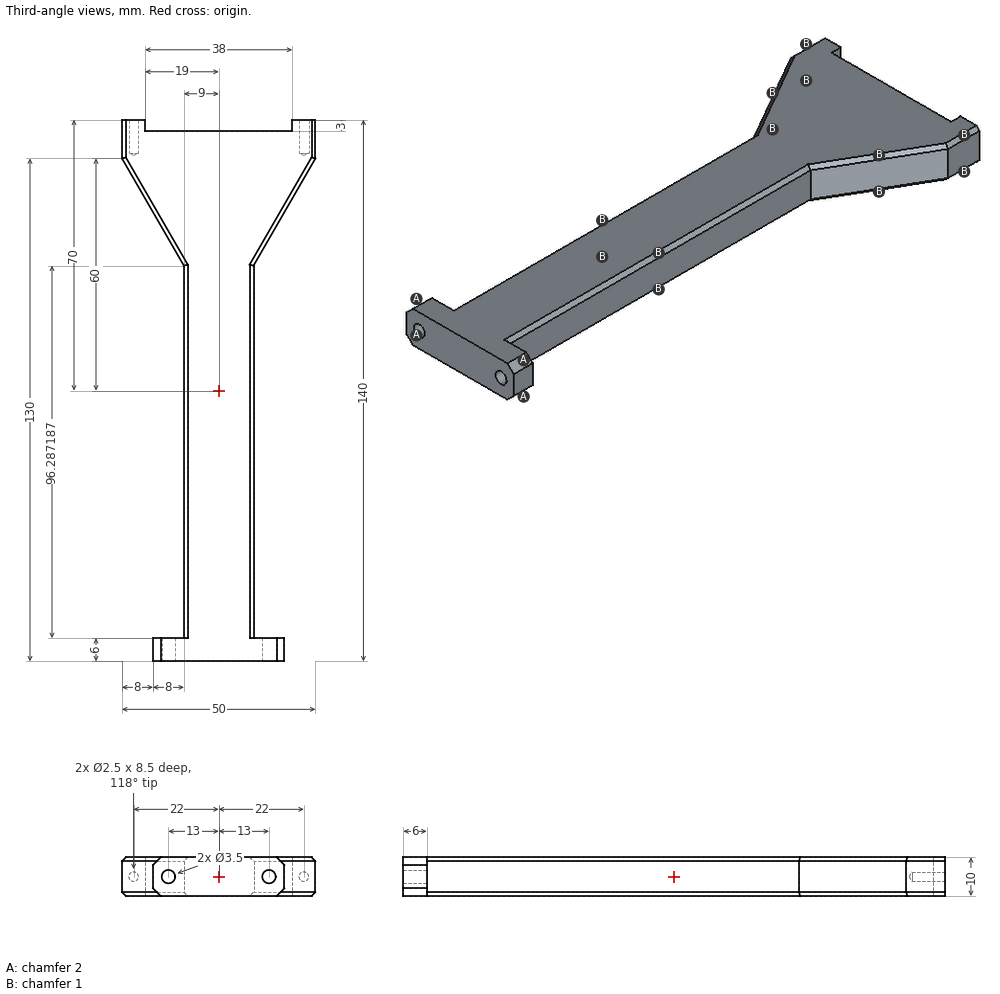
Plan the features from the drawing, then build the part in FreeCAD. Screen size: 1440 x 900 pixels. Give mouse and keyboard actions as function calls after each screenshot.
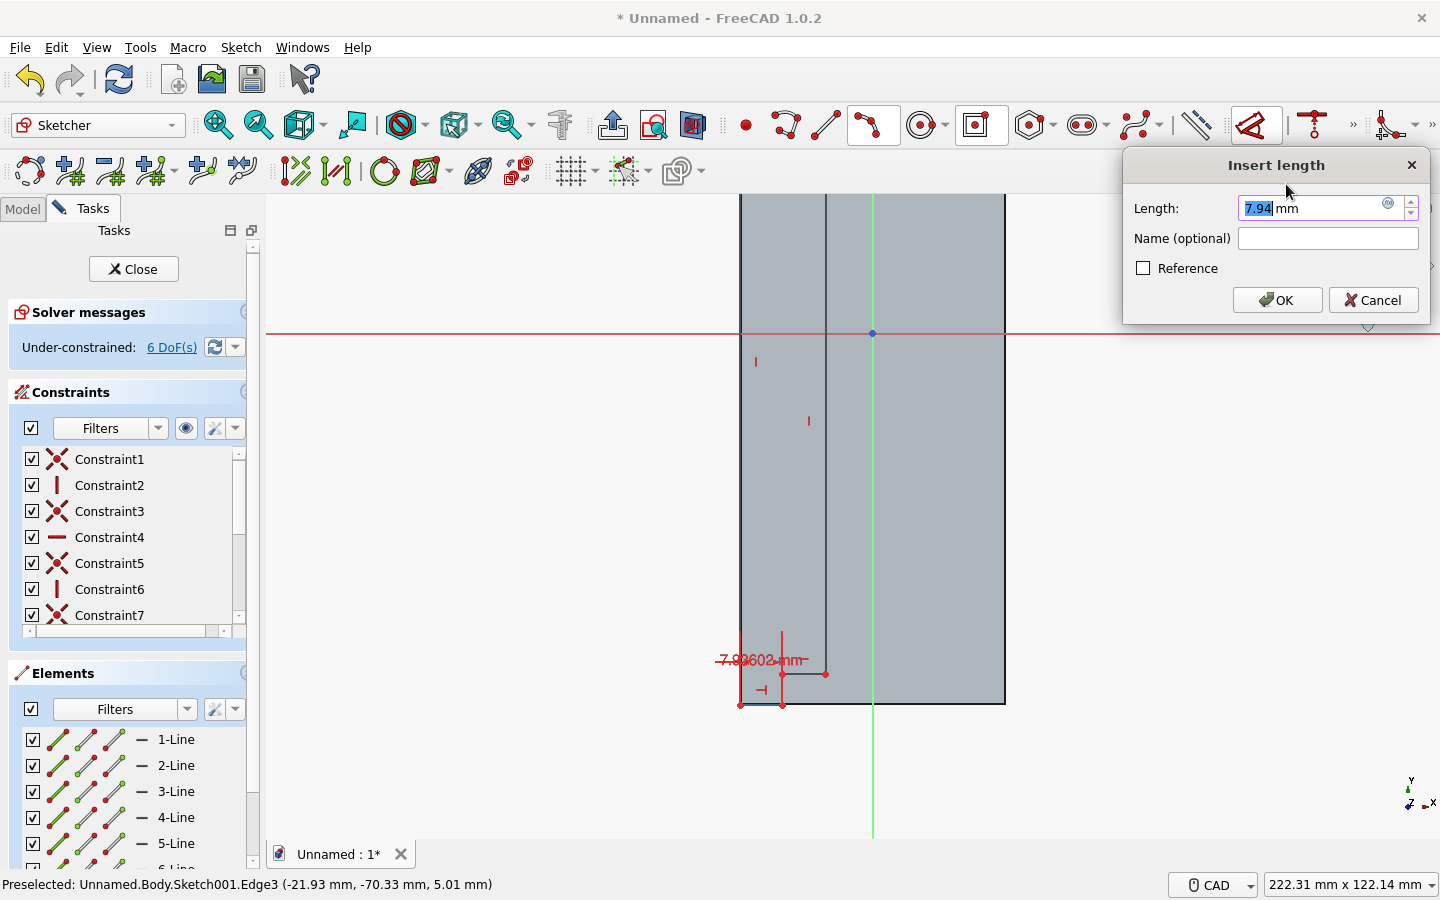
text(8)
key(Return)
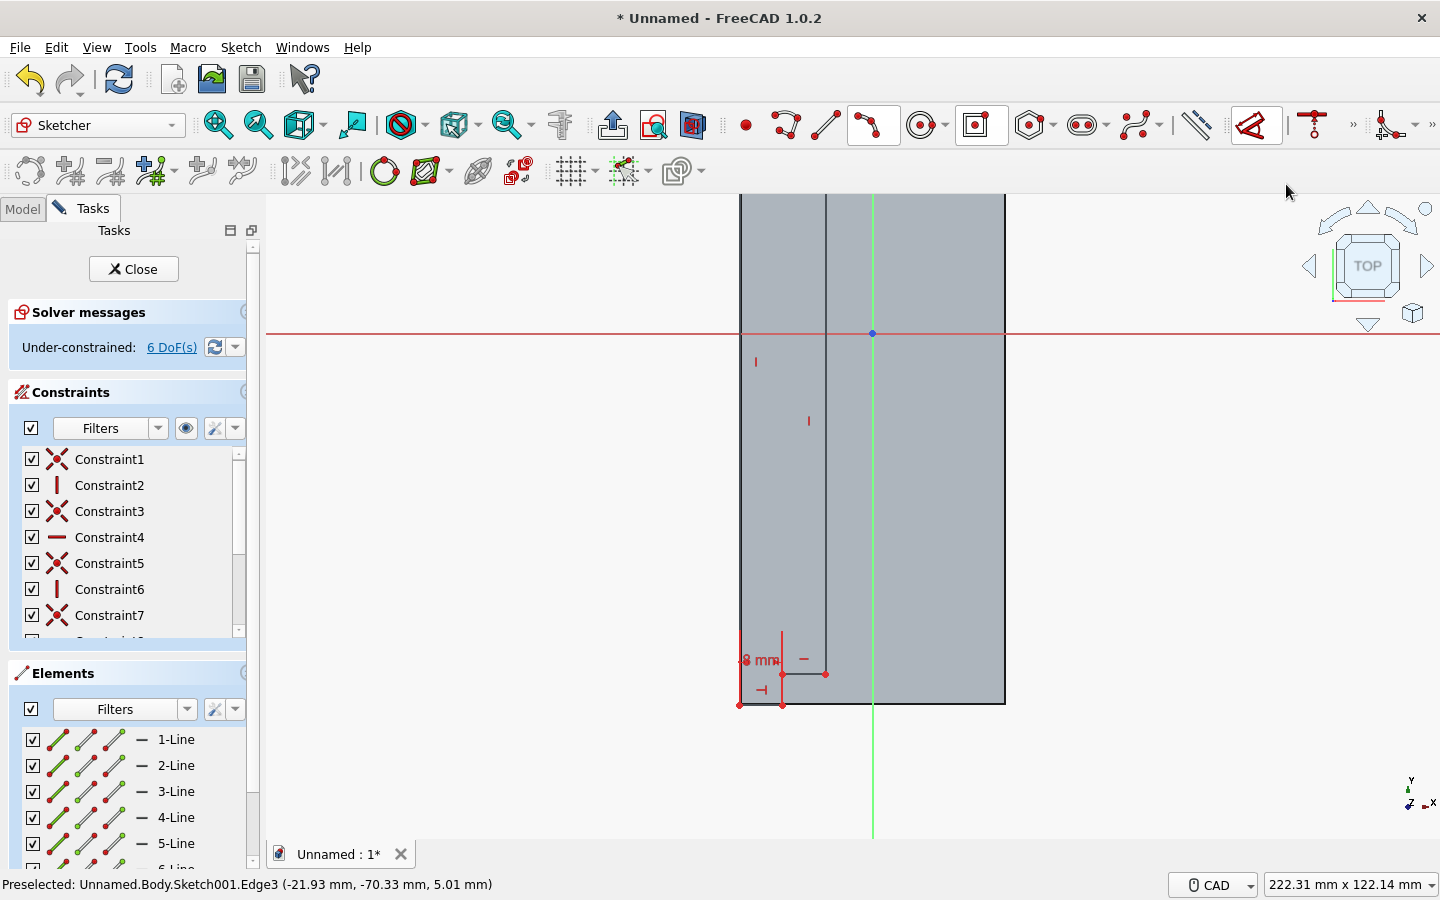
scroll(782, 696, up, 2)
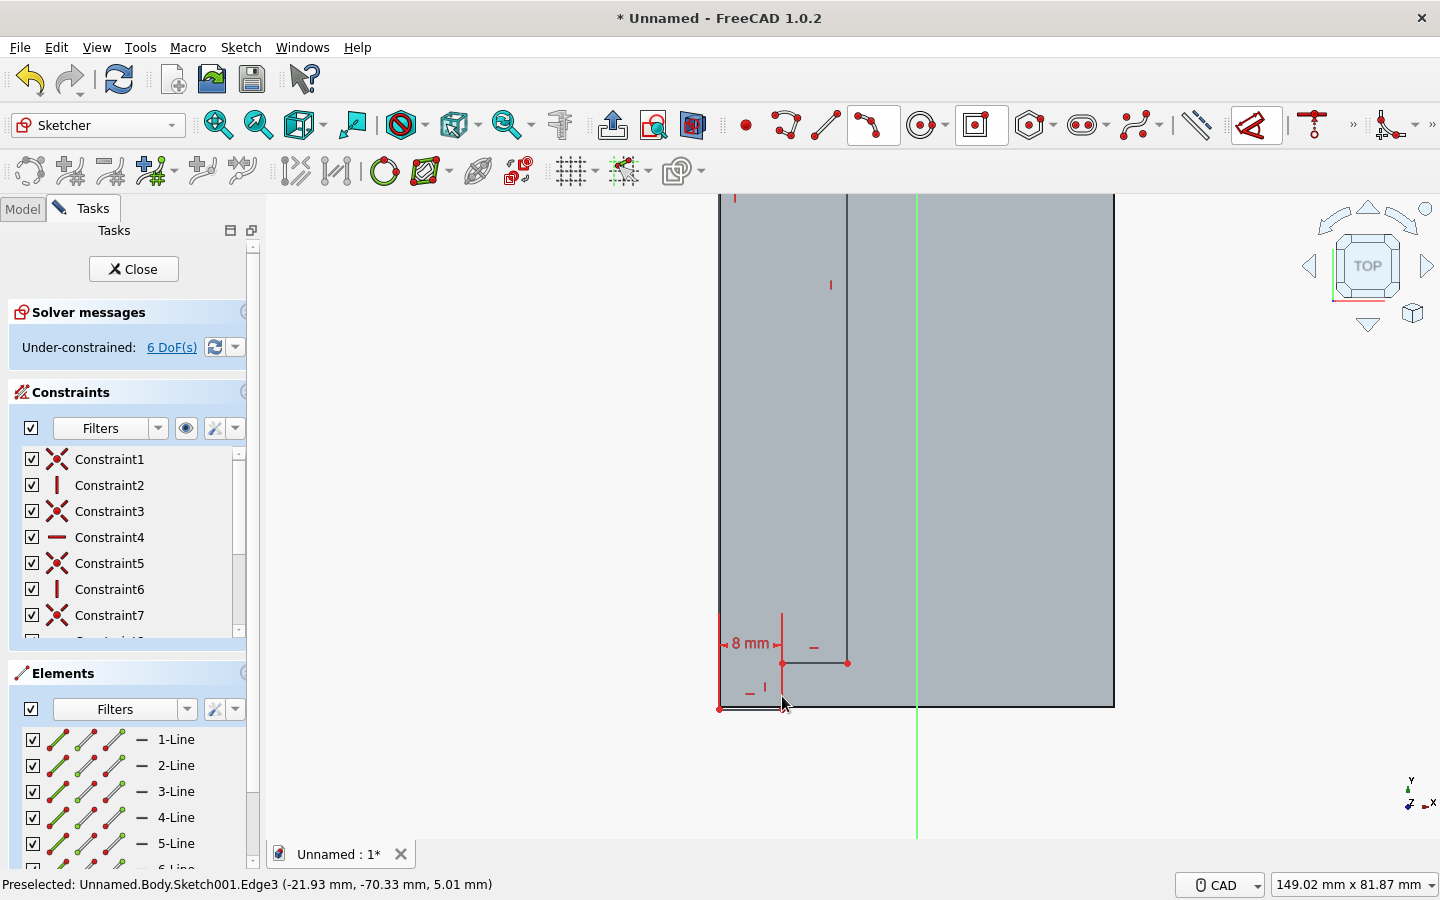
click(782, 696)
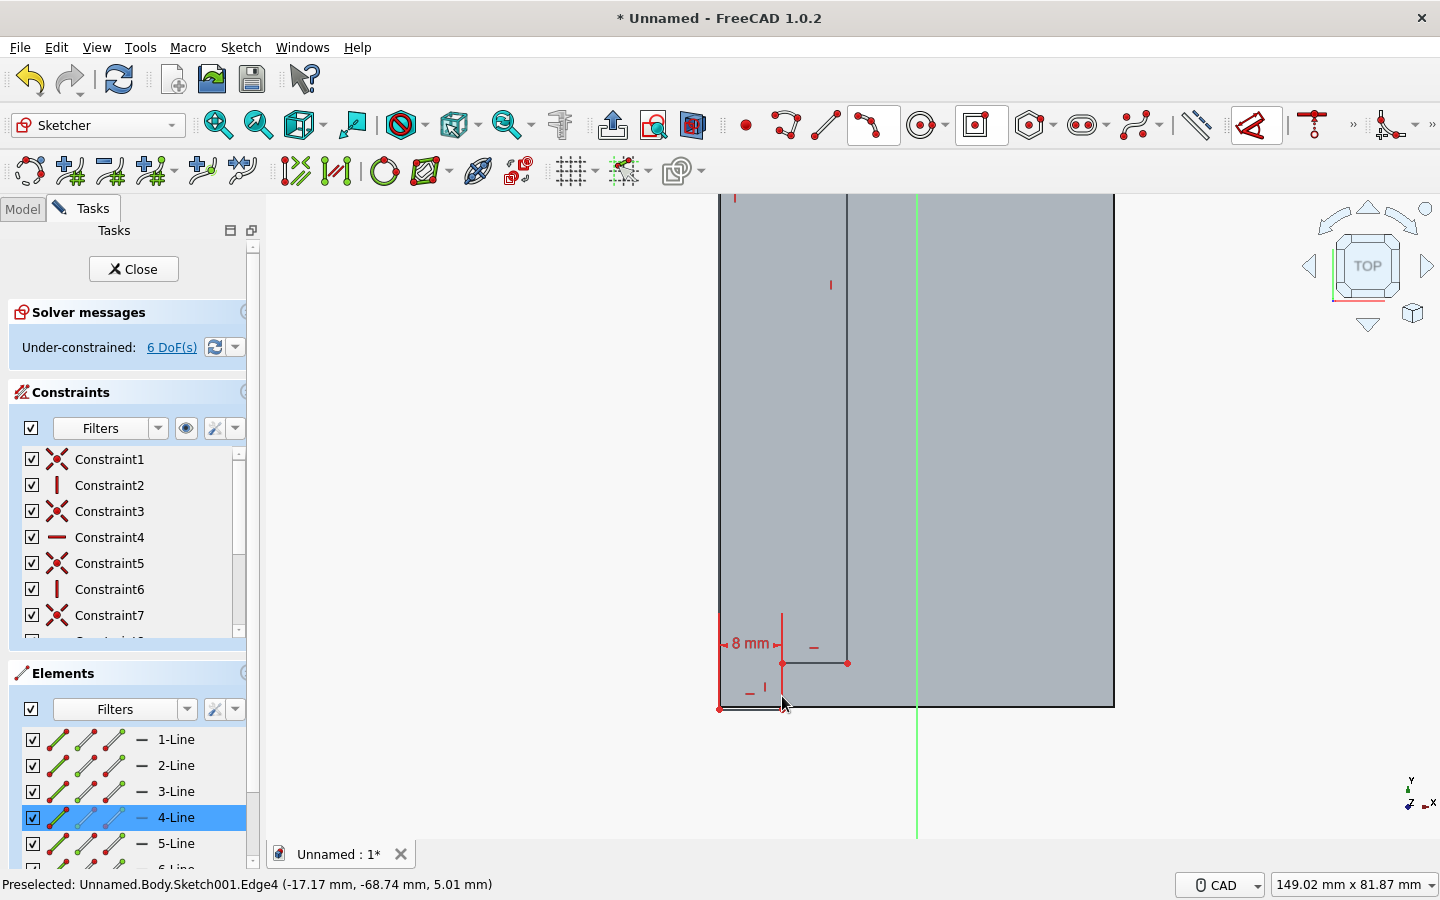
click(1276, 126)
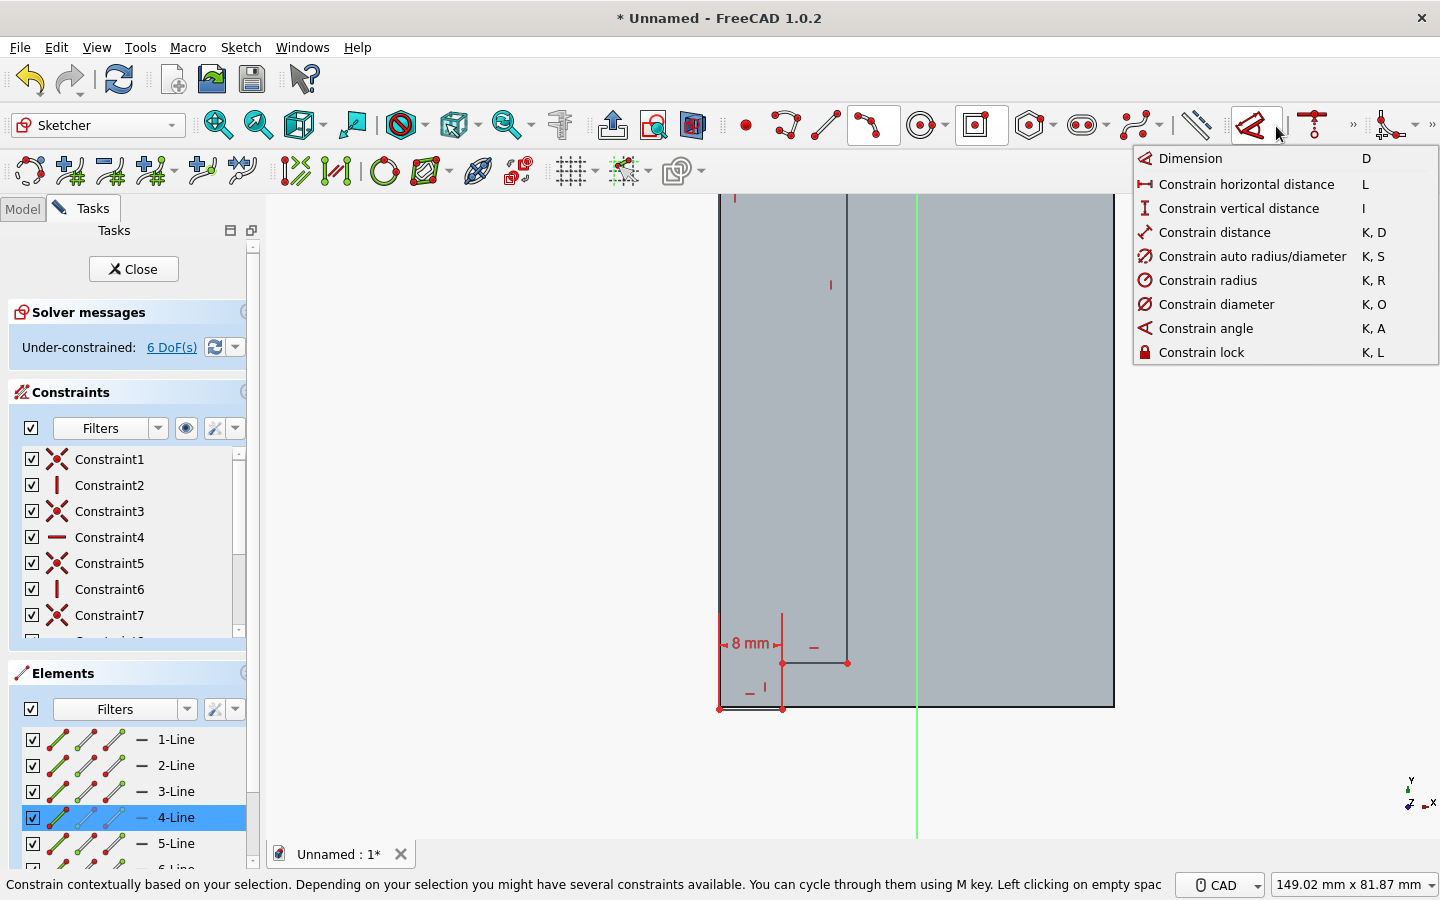
click(1286, 208)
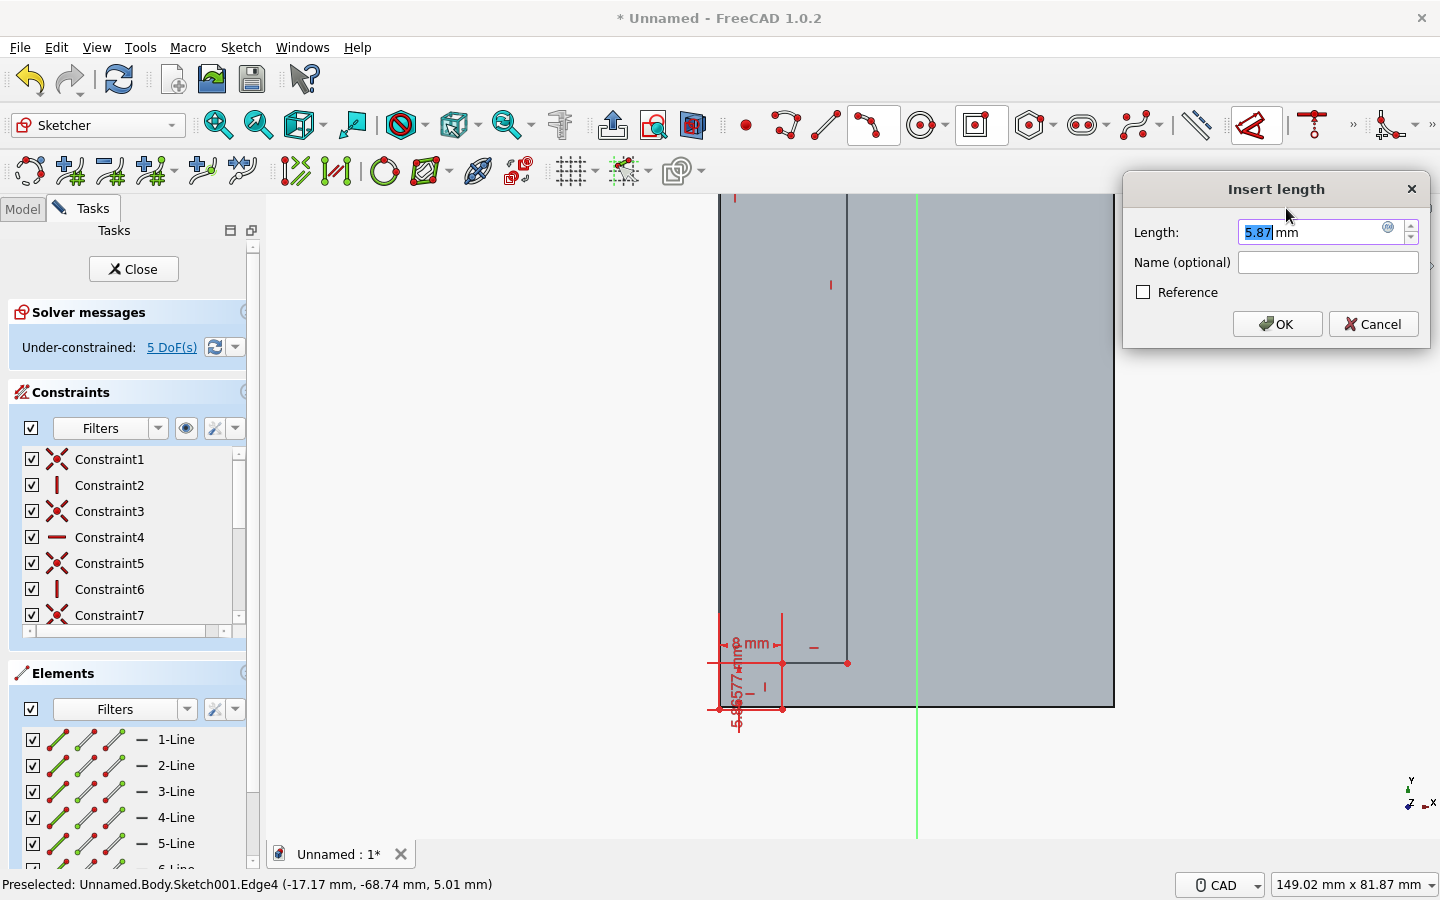
text(6)
key(Return)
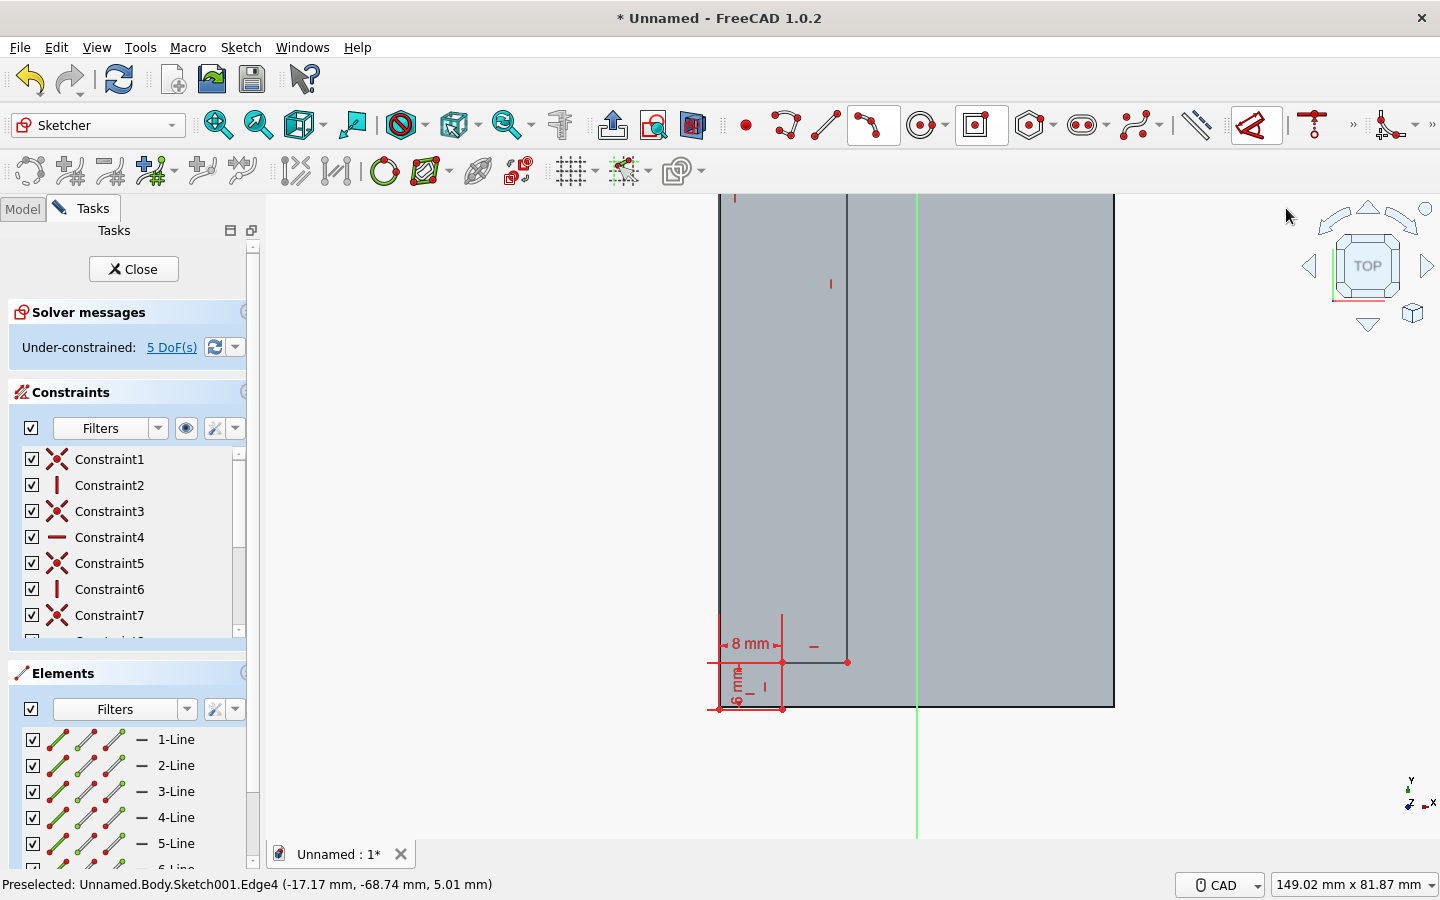
click(802, 663)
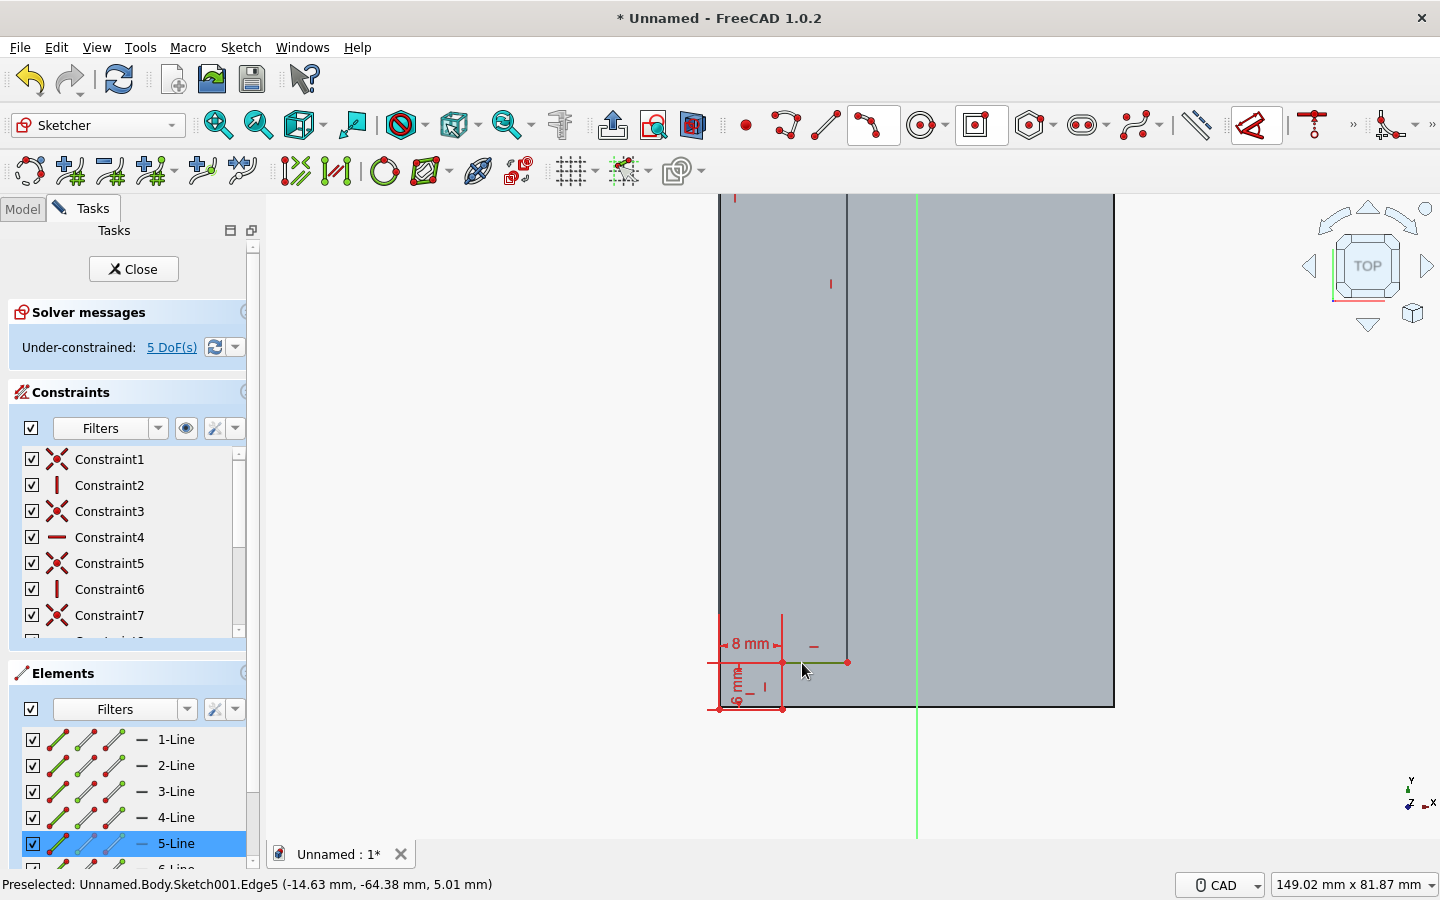
key(l)